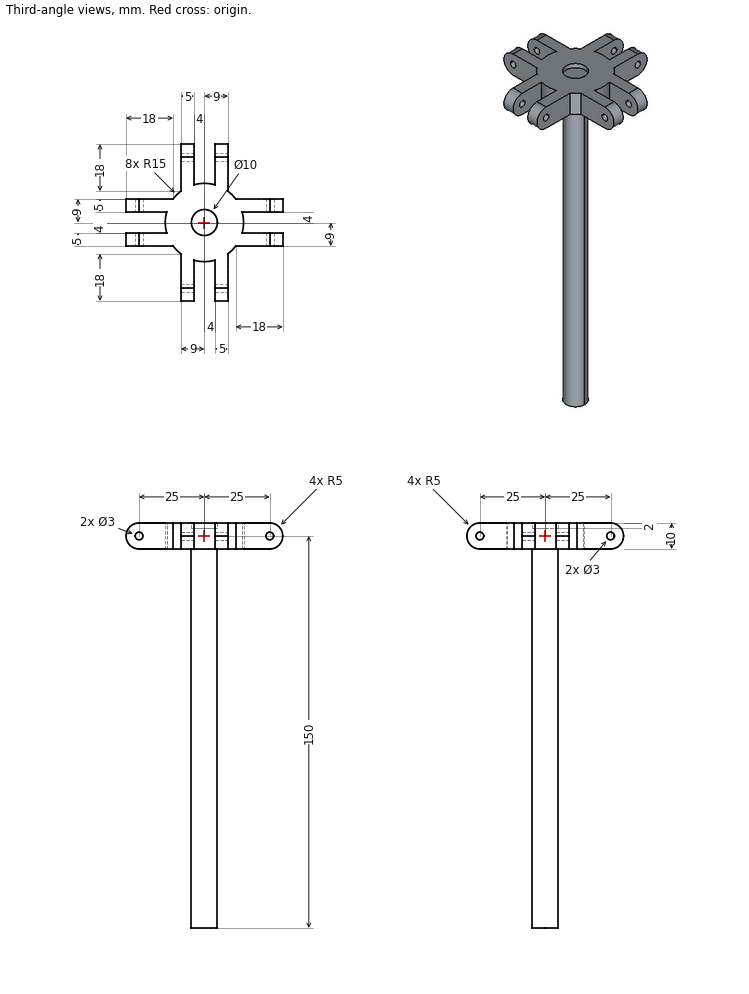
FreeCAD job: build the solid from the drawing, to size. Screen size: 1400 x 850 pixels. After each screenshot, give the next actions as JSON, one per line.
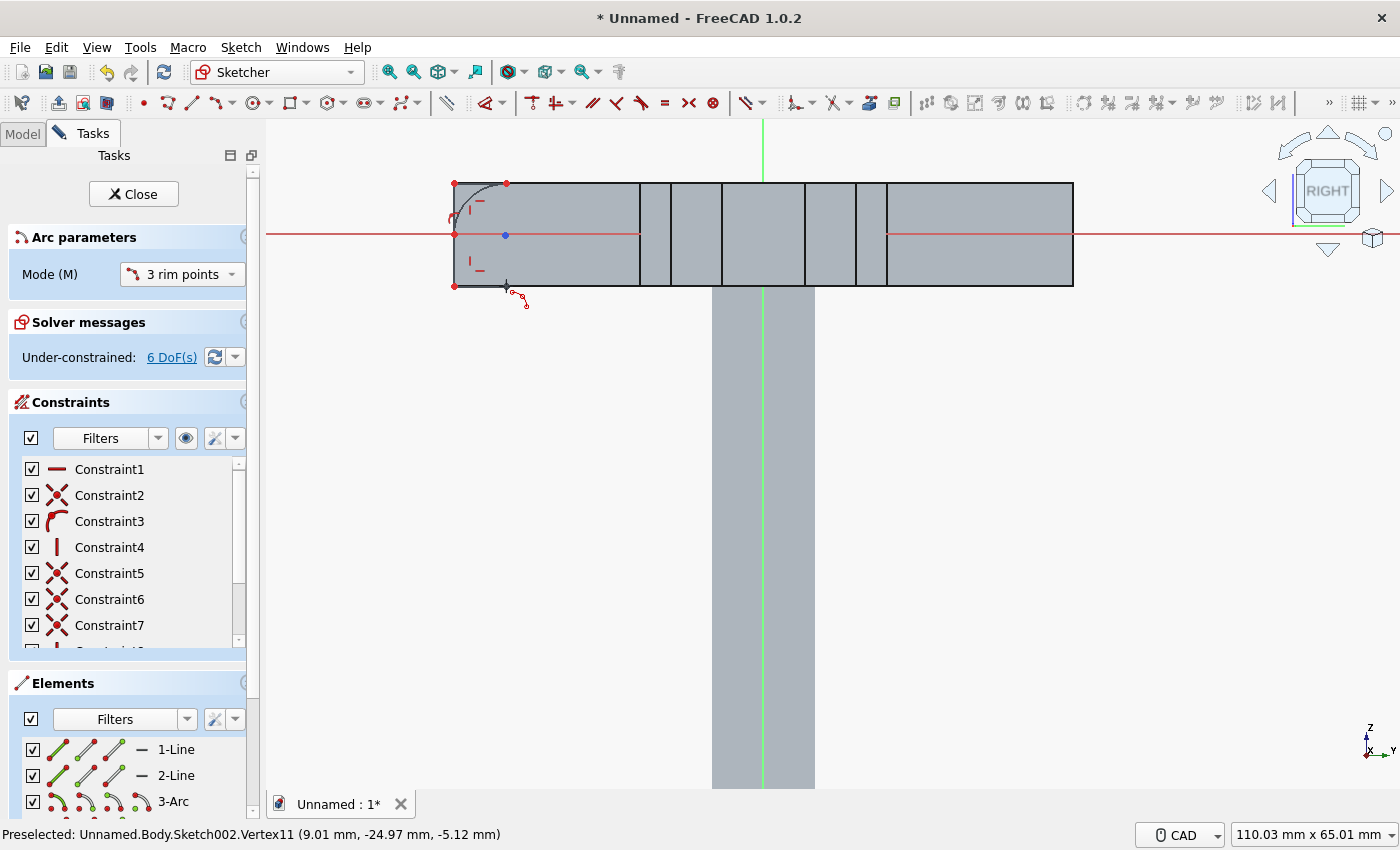
{"action": "left_click", "coordinate": [506, 287]}
{"action": "left_click", "coordinate": [454, 234]}
{"action": "left_click", "coordinate": [469, 271]}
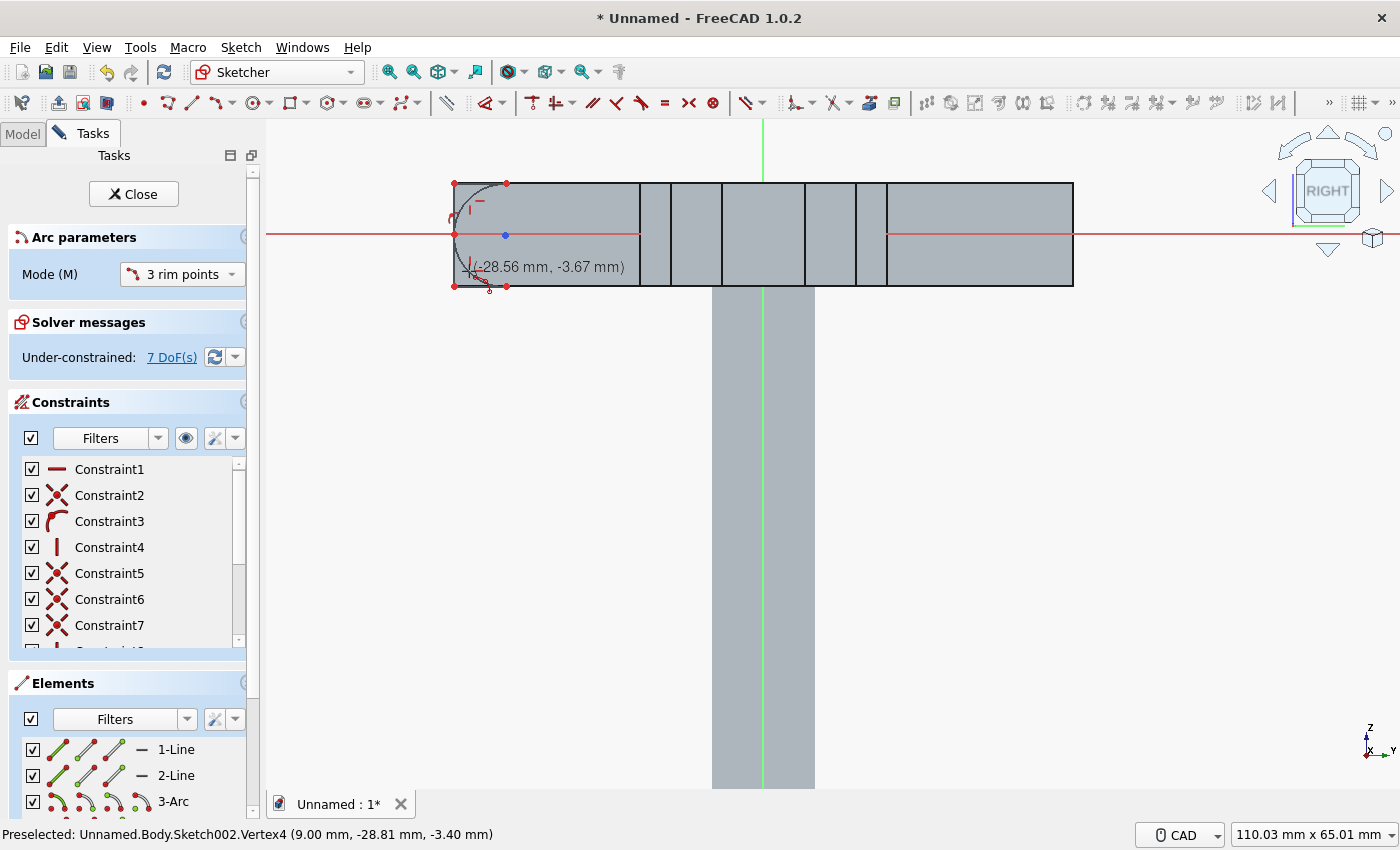
{"action": "key", "text": "g m"}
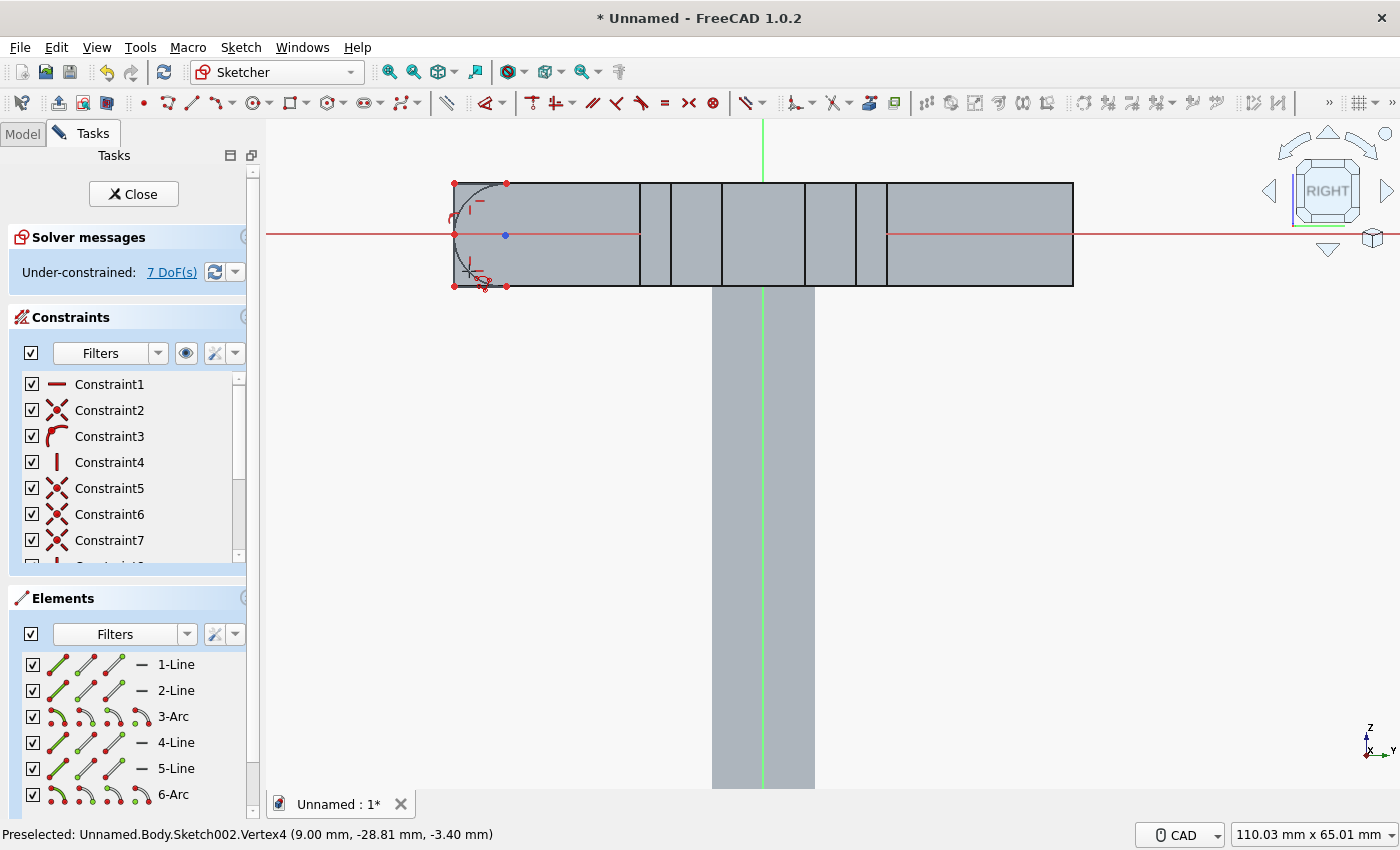
{"action": "left_click", "coordinate": [1073, 234]}
{"action": "left_click", "coordinate": [1073, 183]}
{"action": "left_click", "coordinate": [1021, 183]}
{"action": "right_click", "coordinate": [1021, 183]}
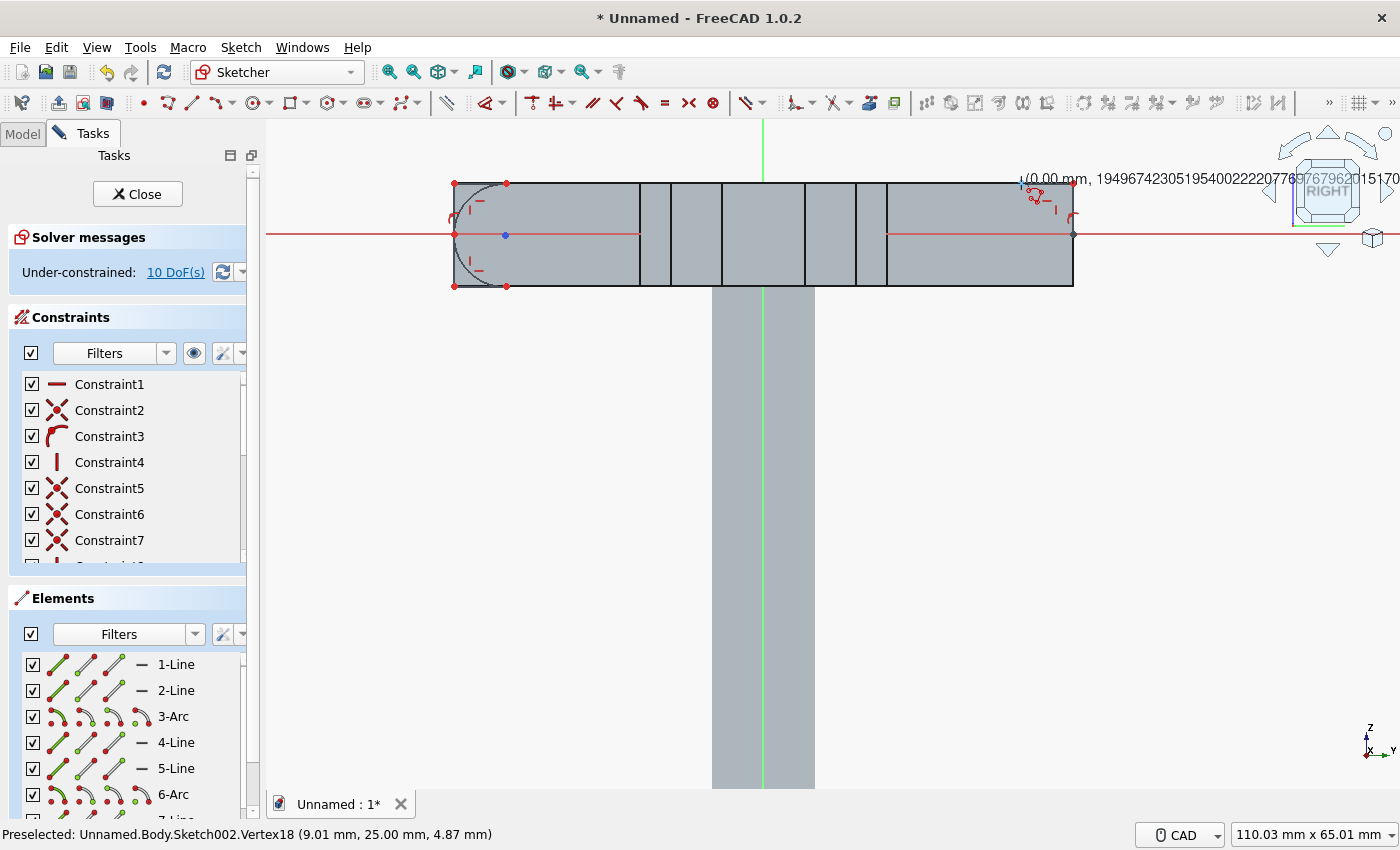
{"action": "left_click", "coordinate": [216, 104]}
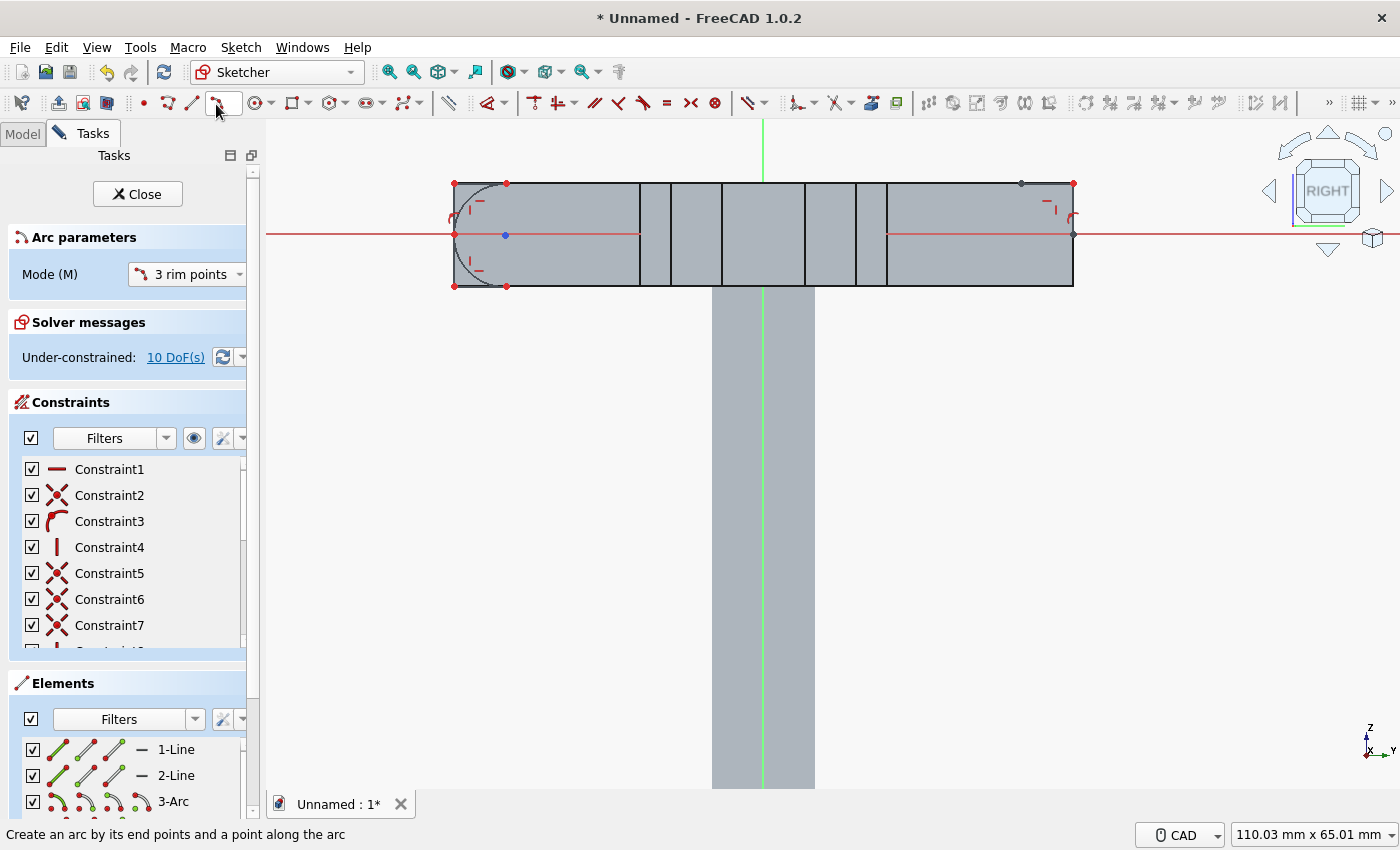
{"action": "left_click", "coordinate": [1021, 184]}
{"action": "left_click", "coordinate": [1073, 234]}
{"action": "left_click", "coordinate": [1057, 198]}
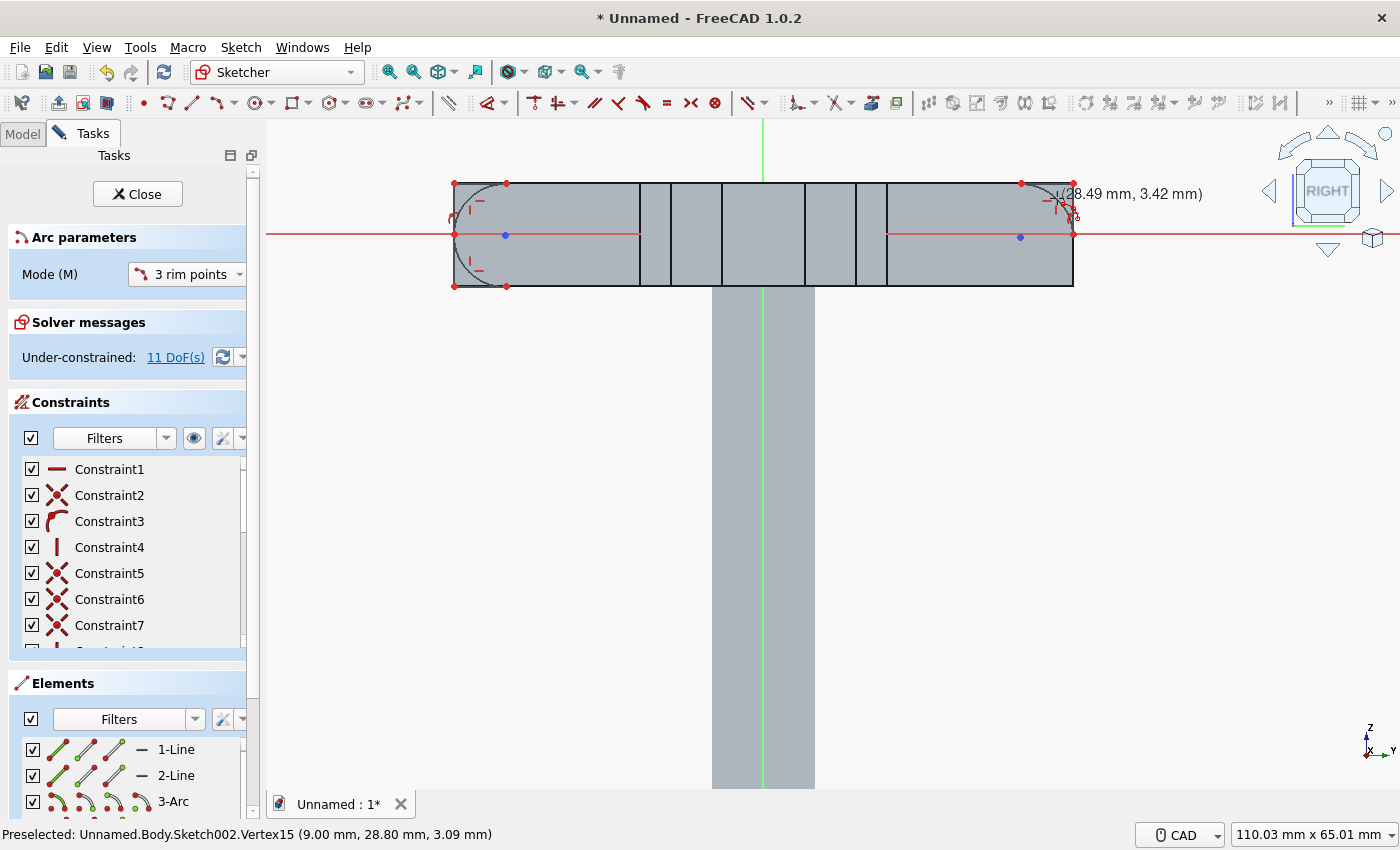
{"action": "key", "text": "g m"}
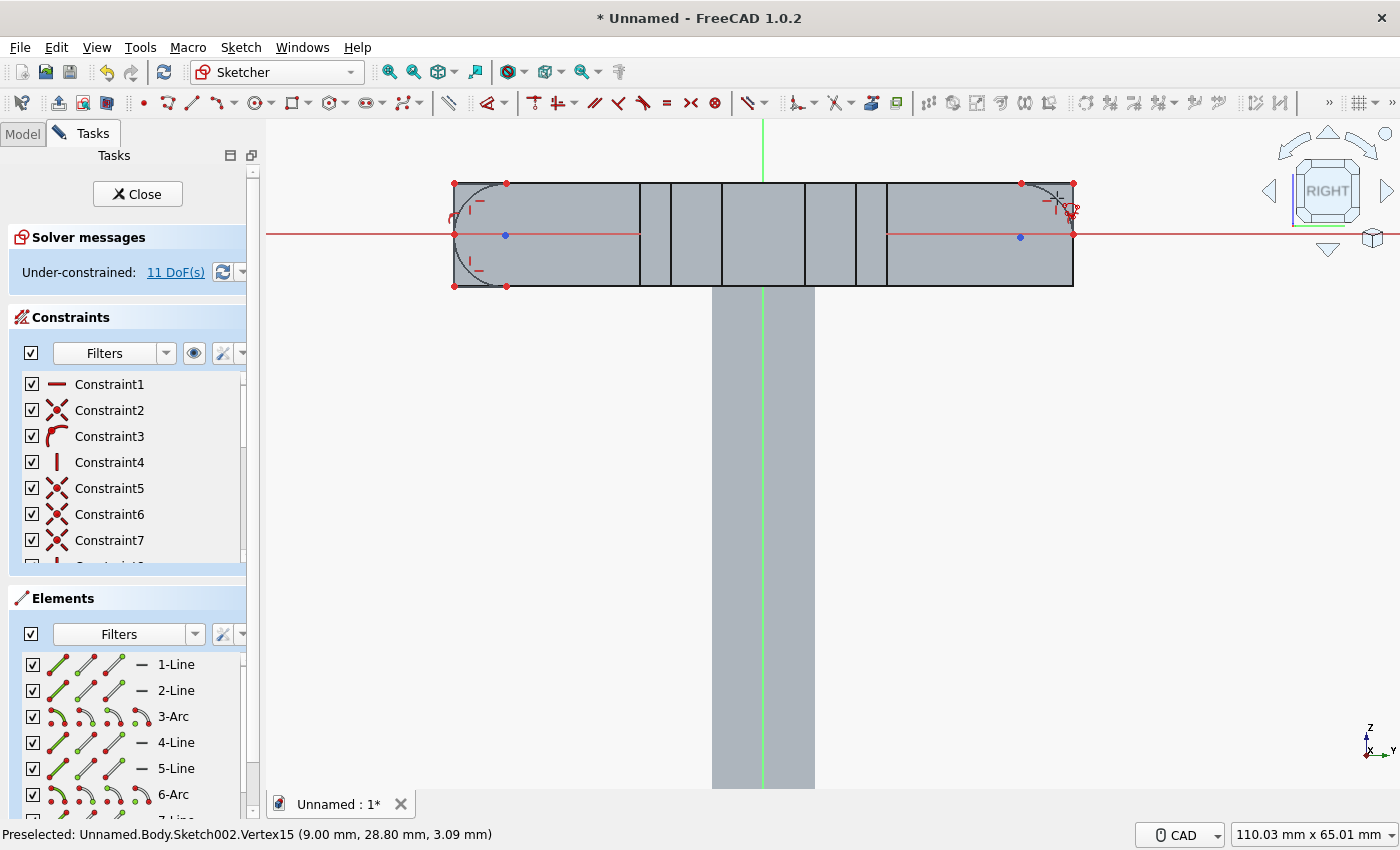
{"action": "left_click", "coordinate": [1021, 286]}
{"action": "left_click", "coordinate": [1073, 286]}
{"action": "left_click", "coordinate": [1073, 234]}
{"action": "right_click", "coordinate": [1073, 286]}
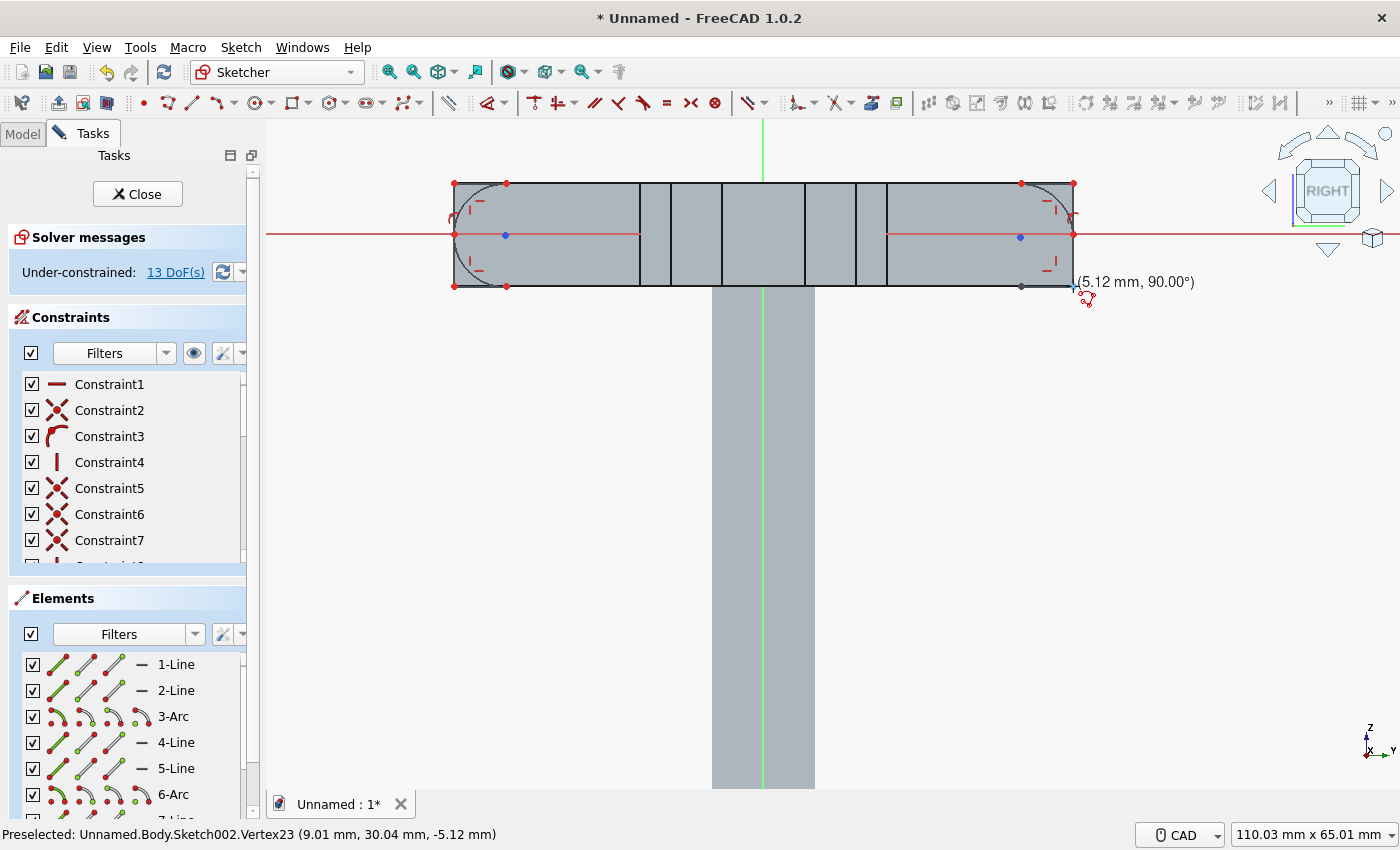
{"action": "key", "text": "g 3 a"}